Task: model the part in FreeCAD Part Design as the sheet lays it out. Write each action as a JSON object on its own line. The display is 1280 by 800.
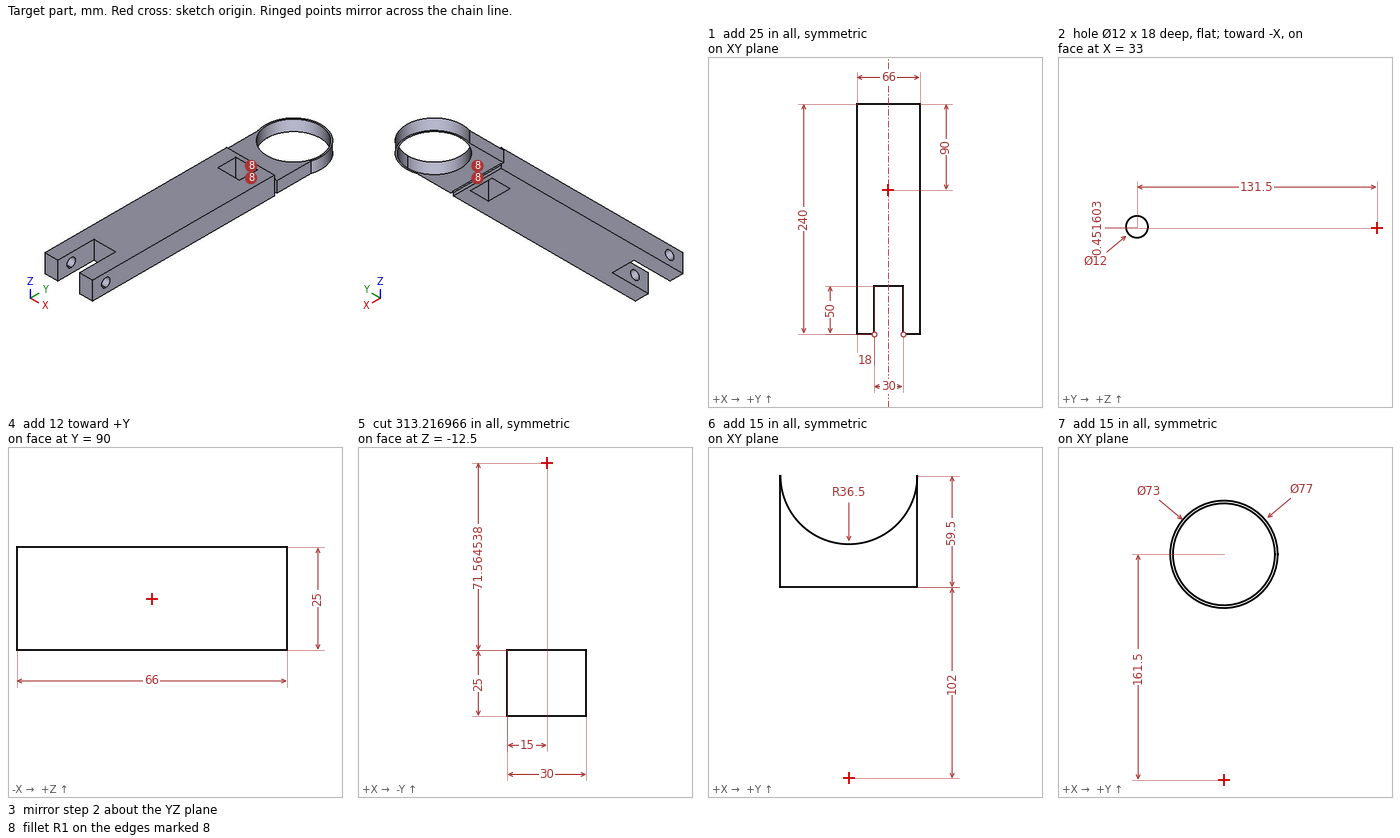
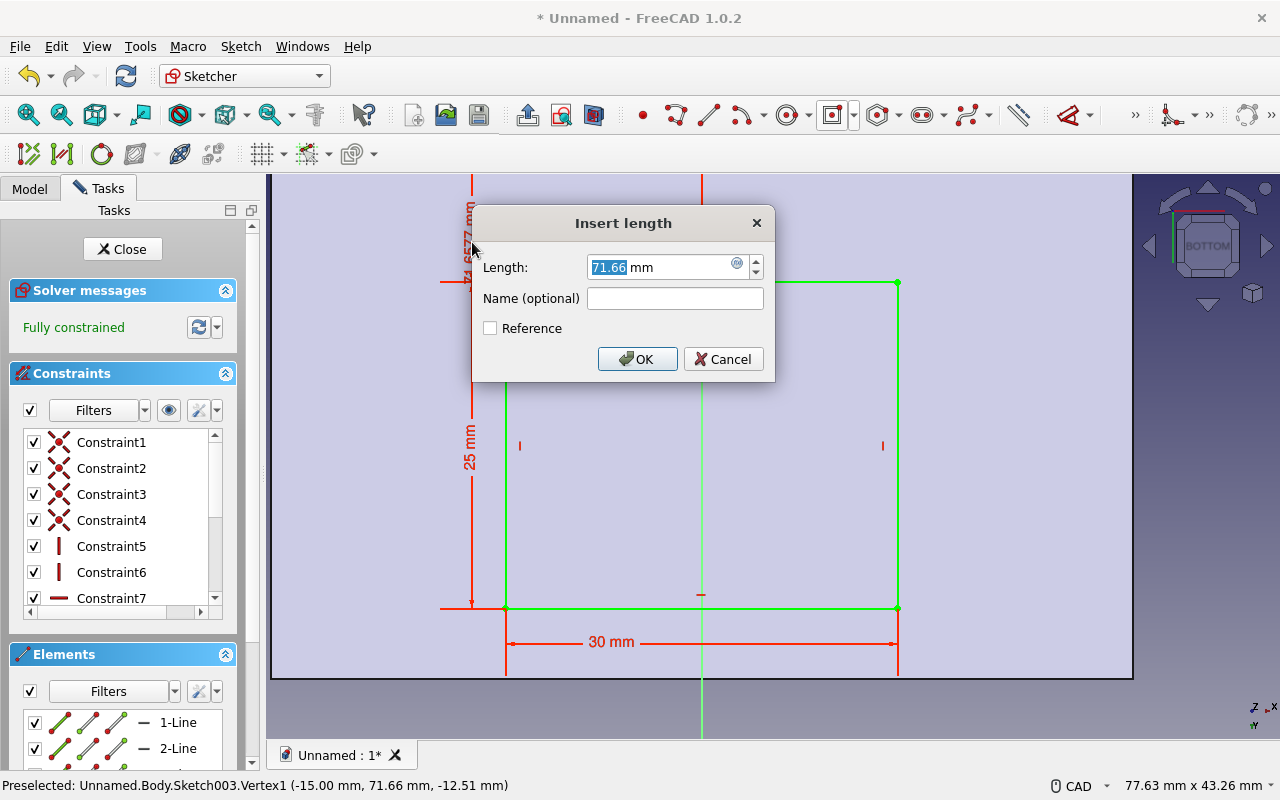
{"action": "type", "text": "71.564538"}
{"action": "key", "text": "Return"}
{"action": "key", "text": "Escape"}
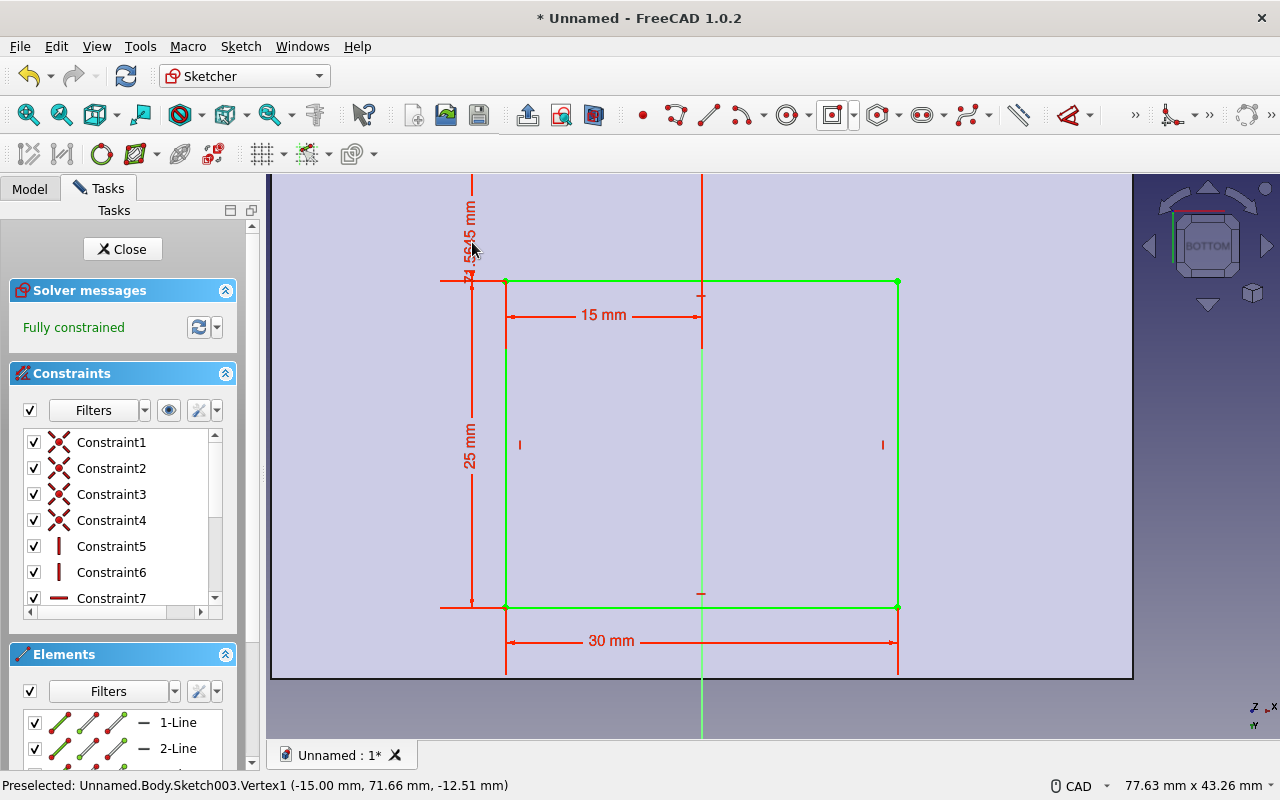
{"action": "left_click", "coordinate": [123, 249]}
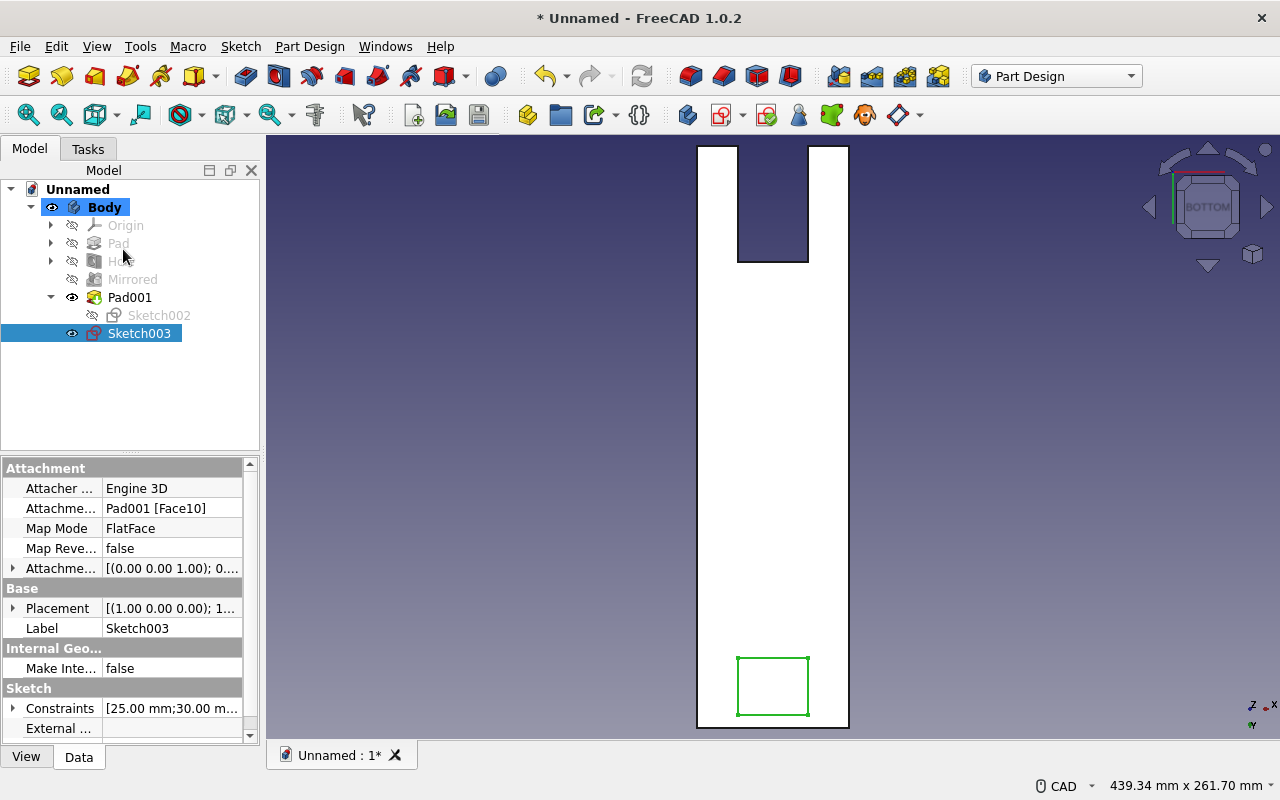
{"action": "left_click", "coordinate": [246, 76]}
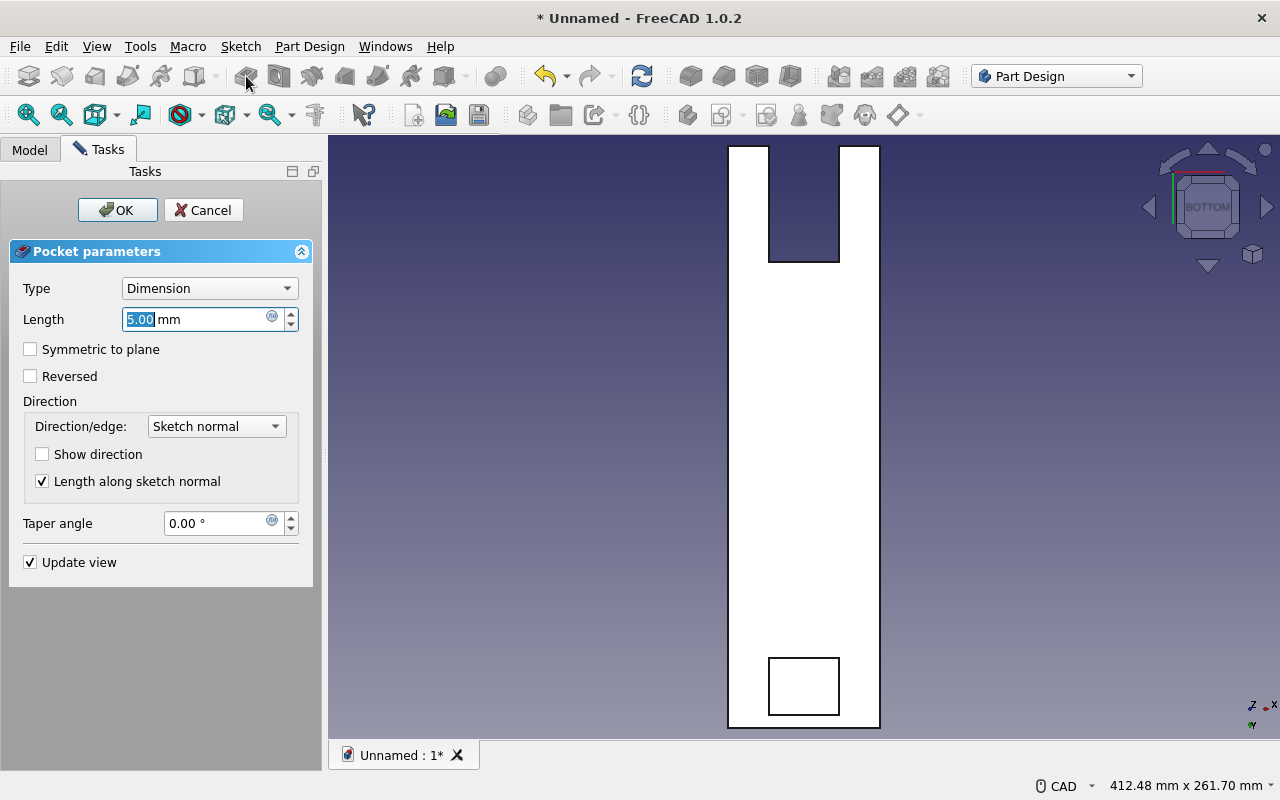
{"action": "type", "text": "313.216966"}
{"action": "key", "text": "Tab"}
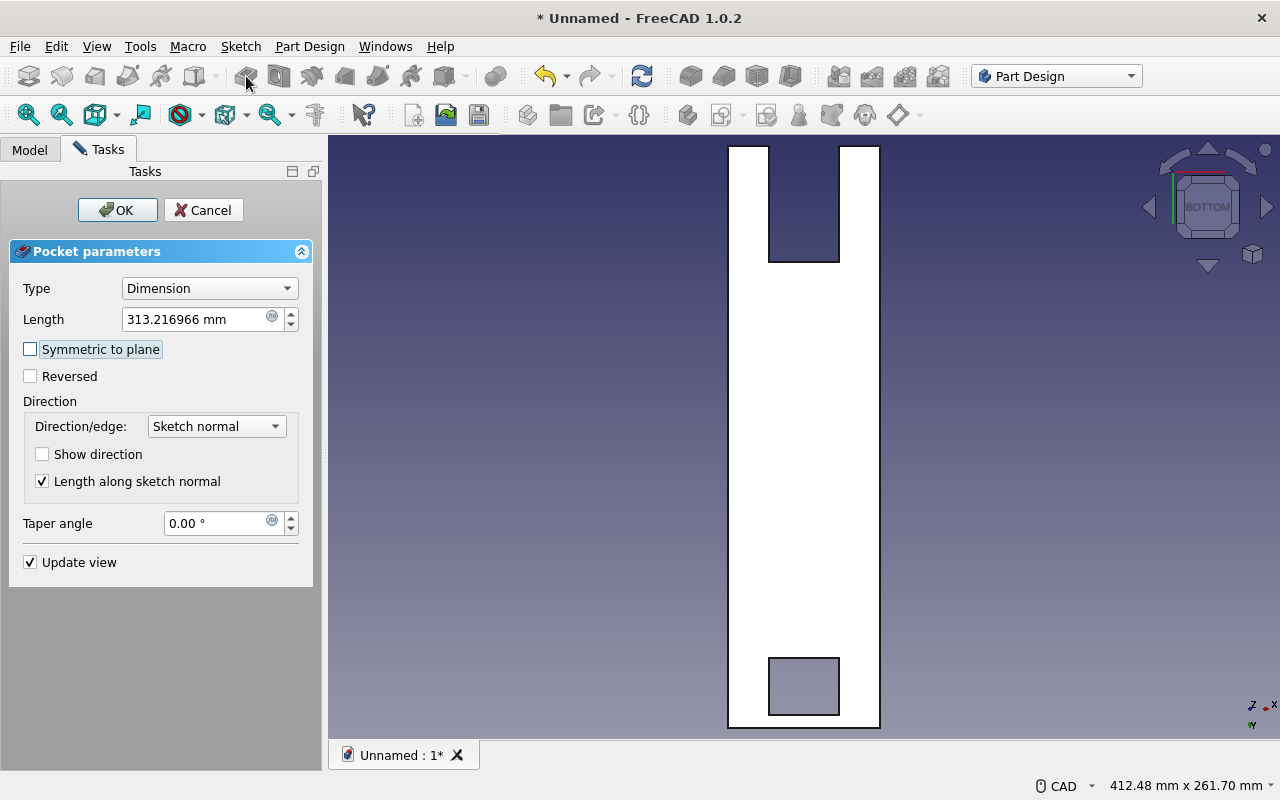
{"action": "left_click", "coordinate": [31, 349]}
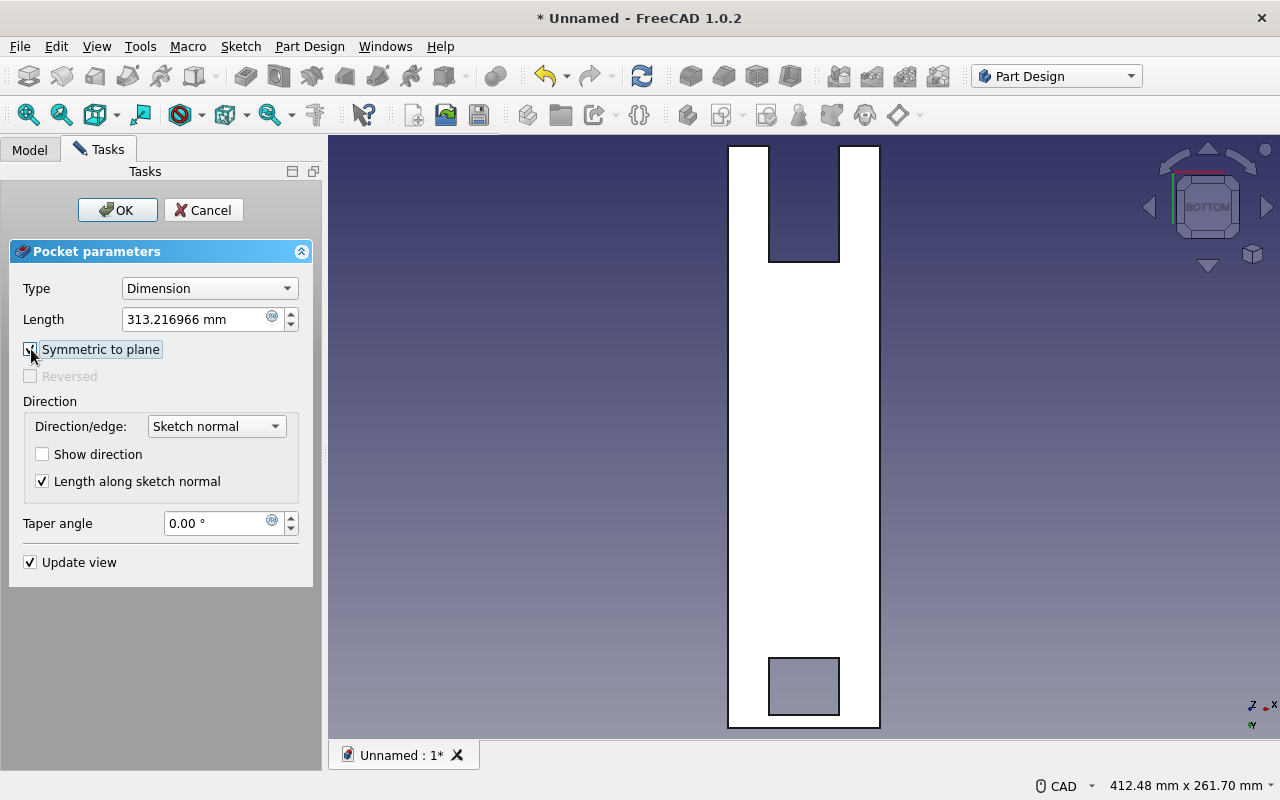
{"action": "left_click", "coordinate": [118, 210]}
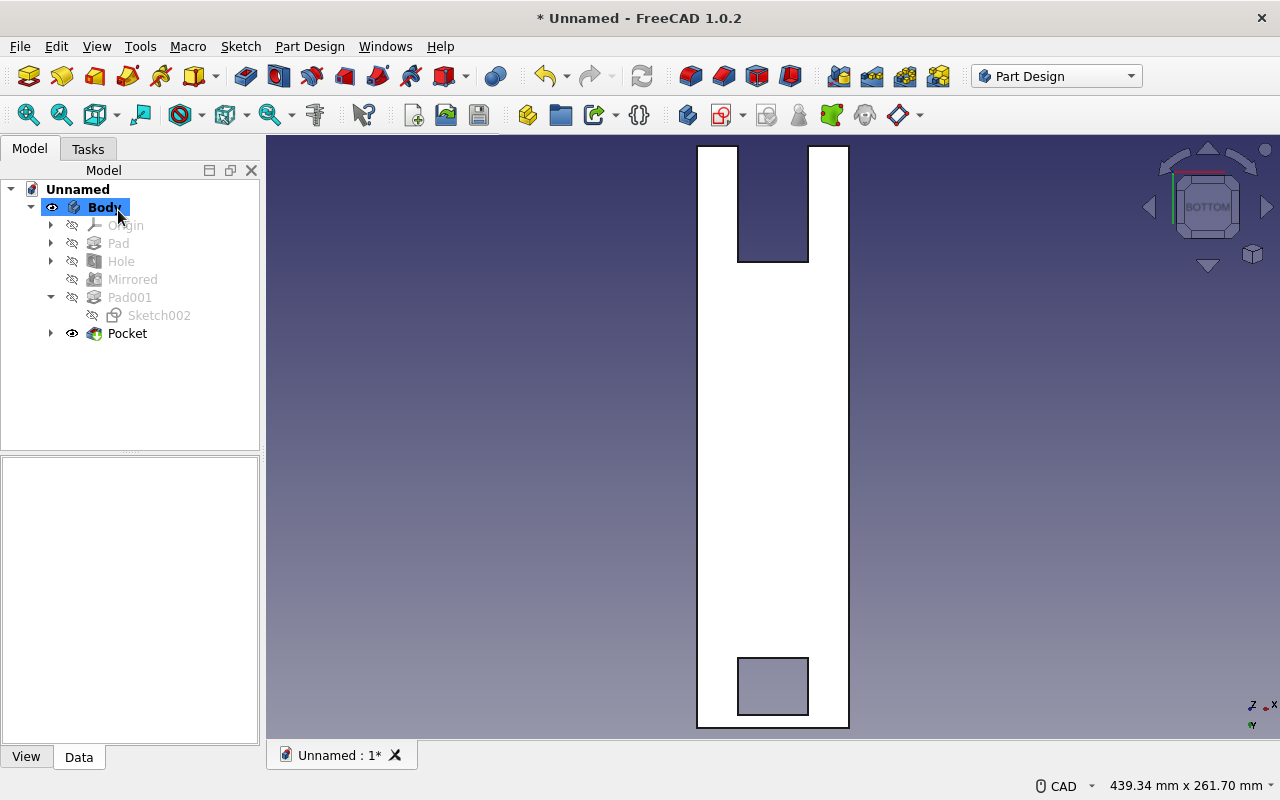
{"action": "left_click", "coordinate": [720, 116]}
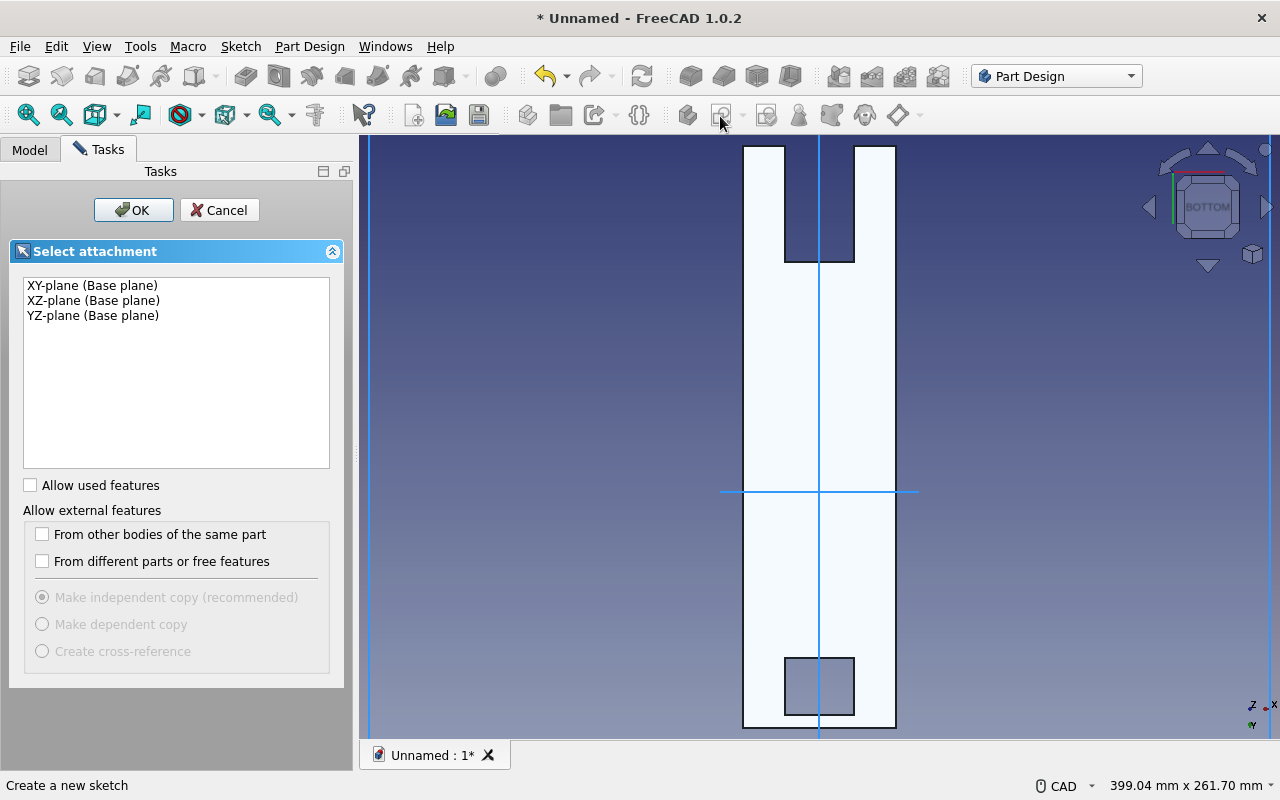
{"action": "left_click", "coordinate": [84, 286]}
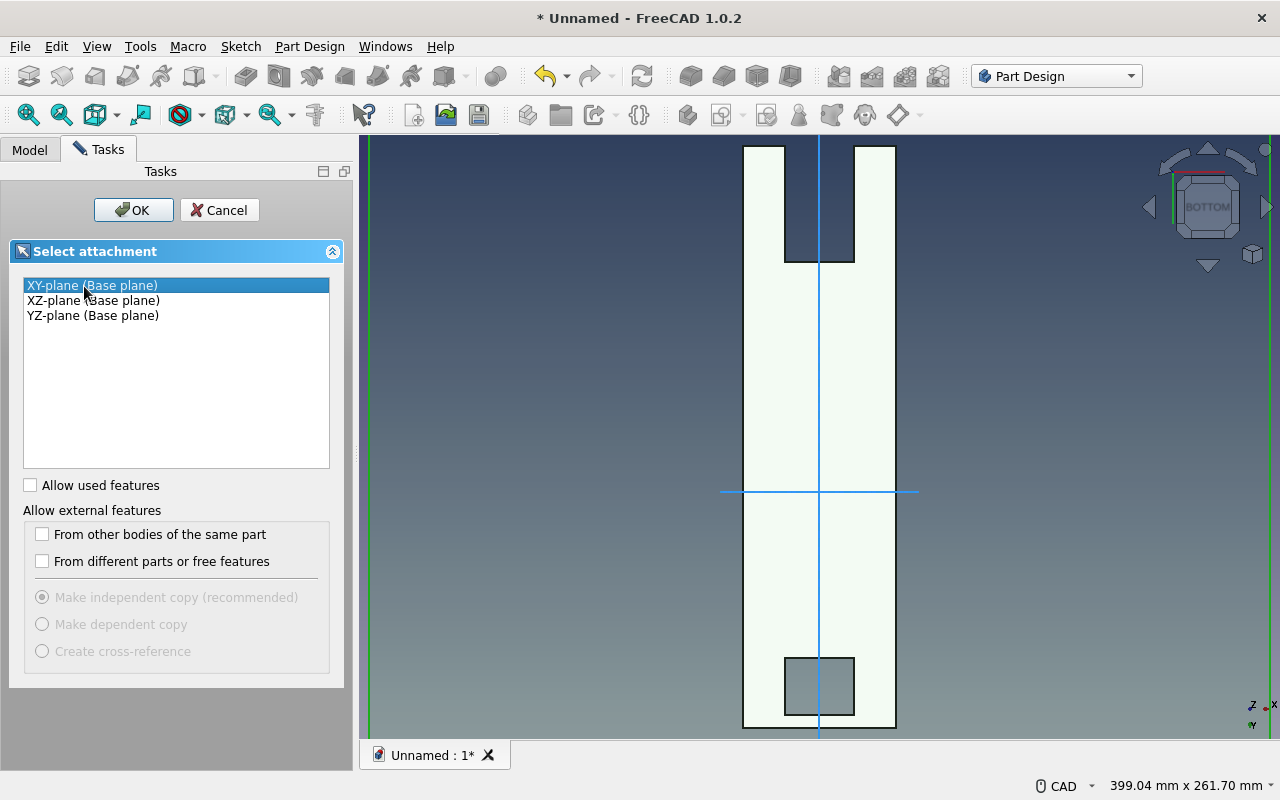
{"action": "left_click", "coordinate": [134, 210]}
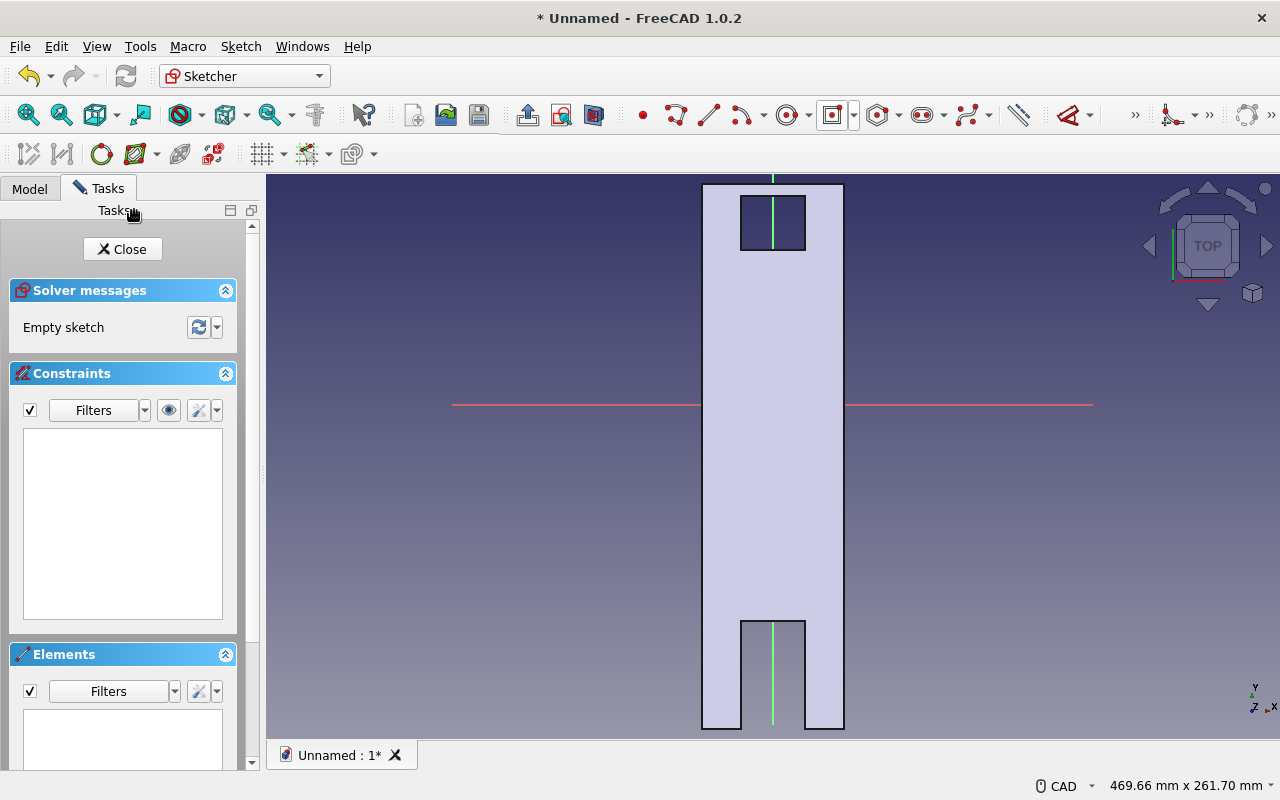
{"action": "key", "text": "q s"}